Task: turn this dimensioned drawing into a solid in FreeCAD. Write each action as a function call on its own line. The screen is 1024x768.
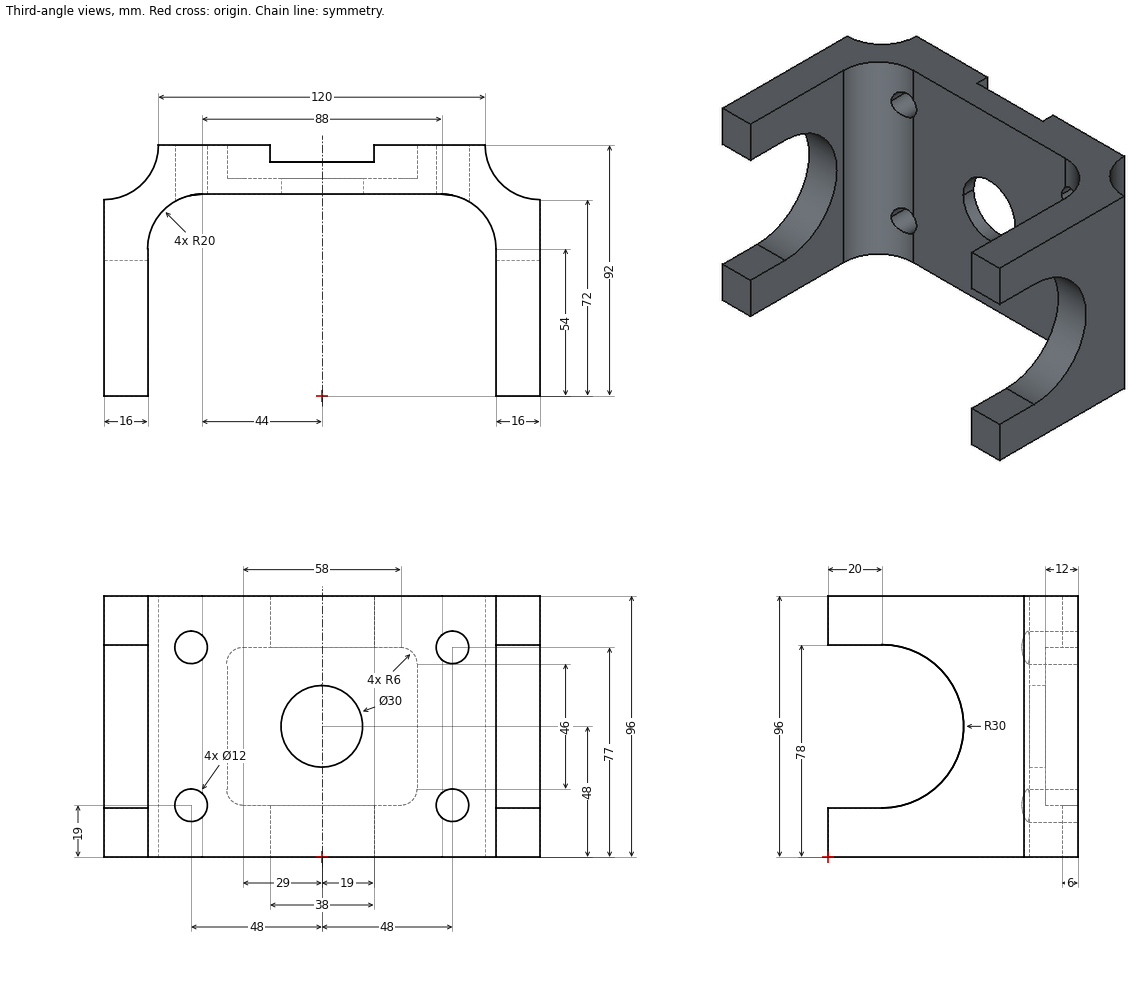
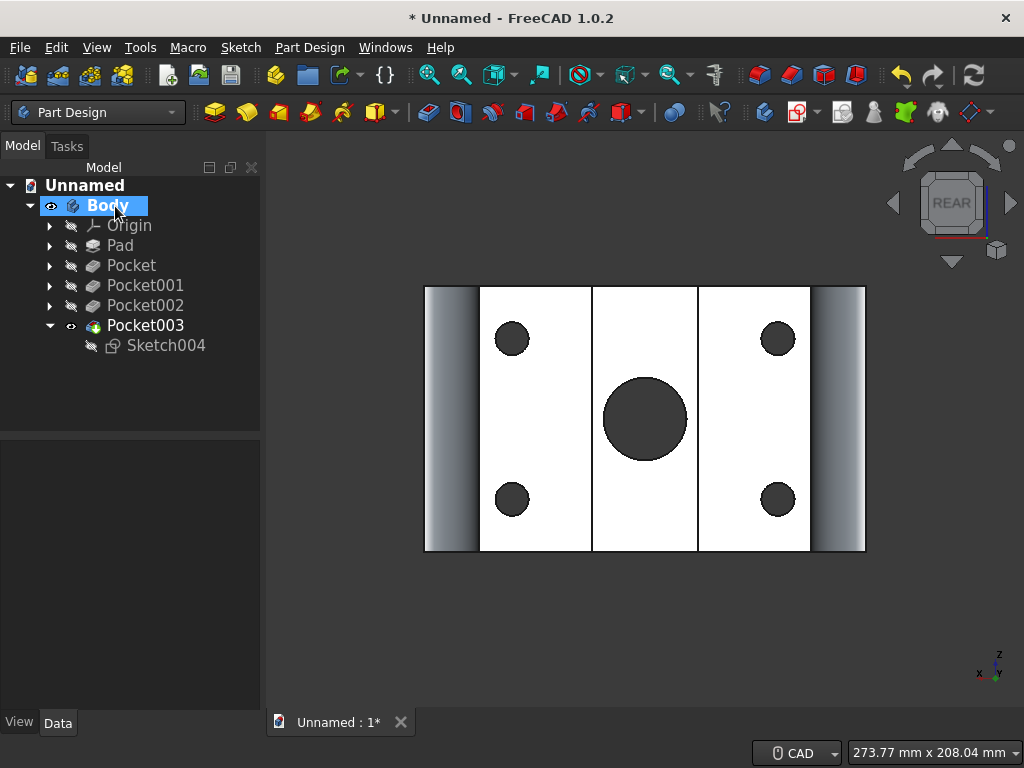
click(536, 418)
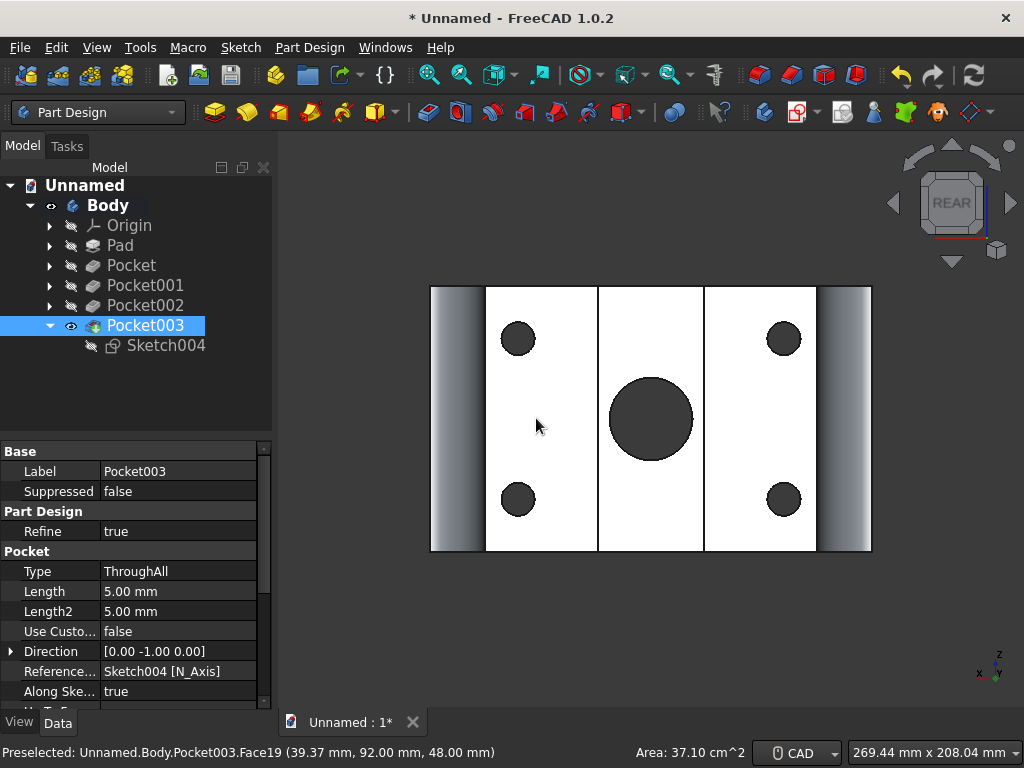
click(798, 112)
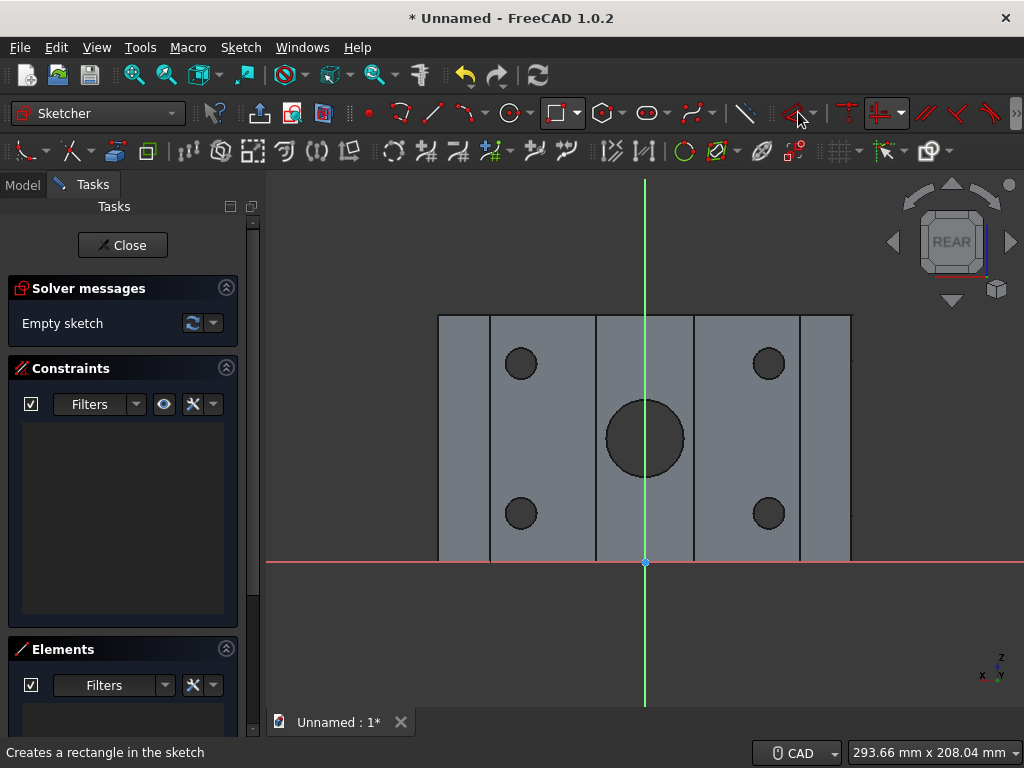
scroll(728, 493, up, 3)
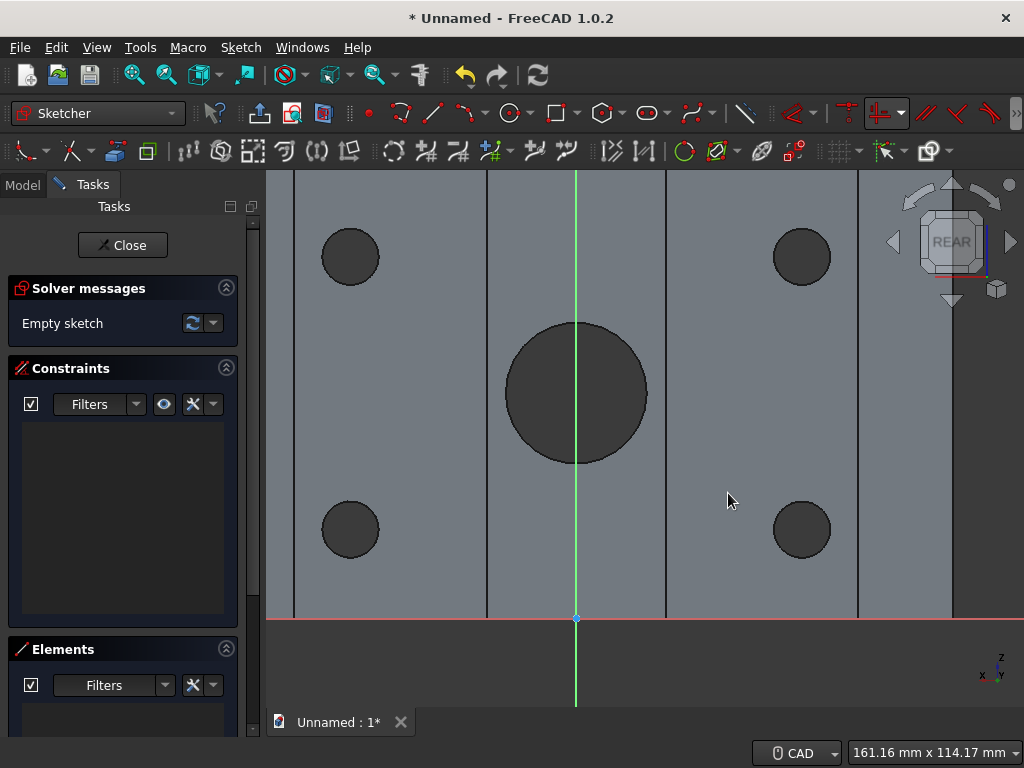
click(434, 114)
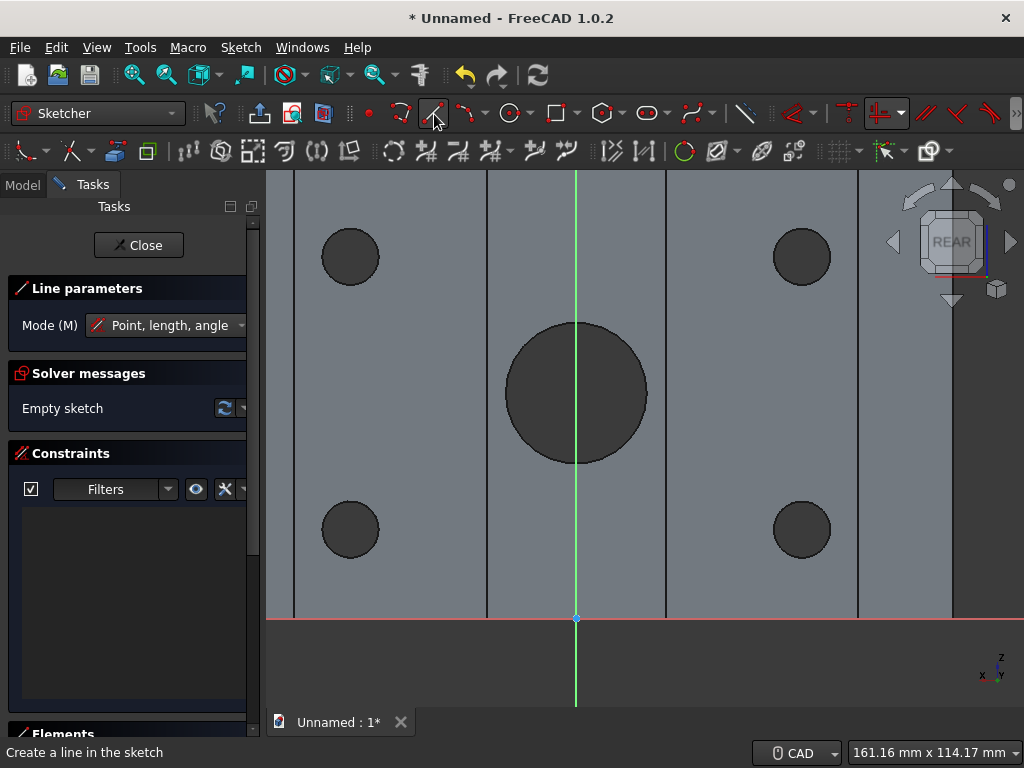
click(713, 257)
click(440, 257)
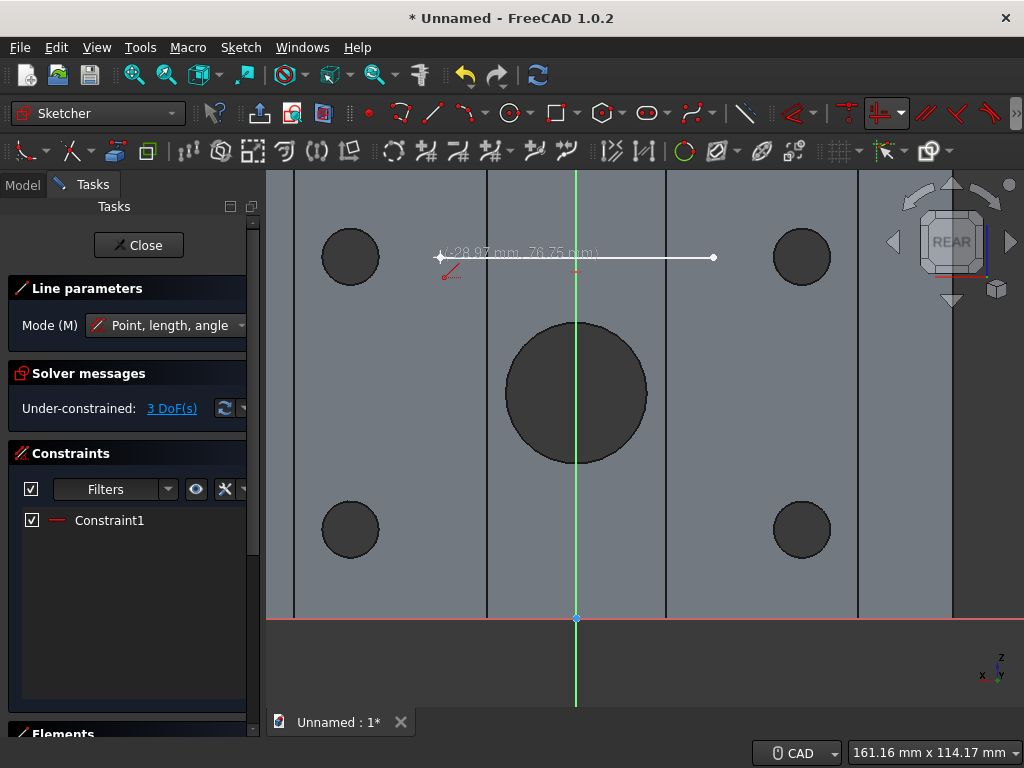
click(412, 285)
click(412, 501)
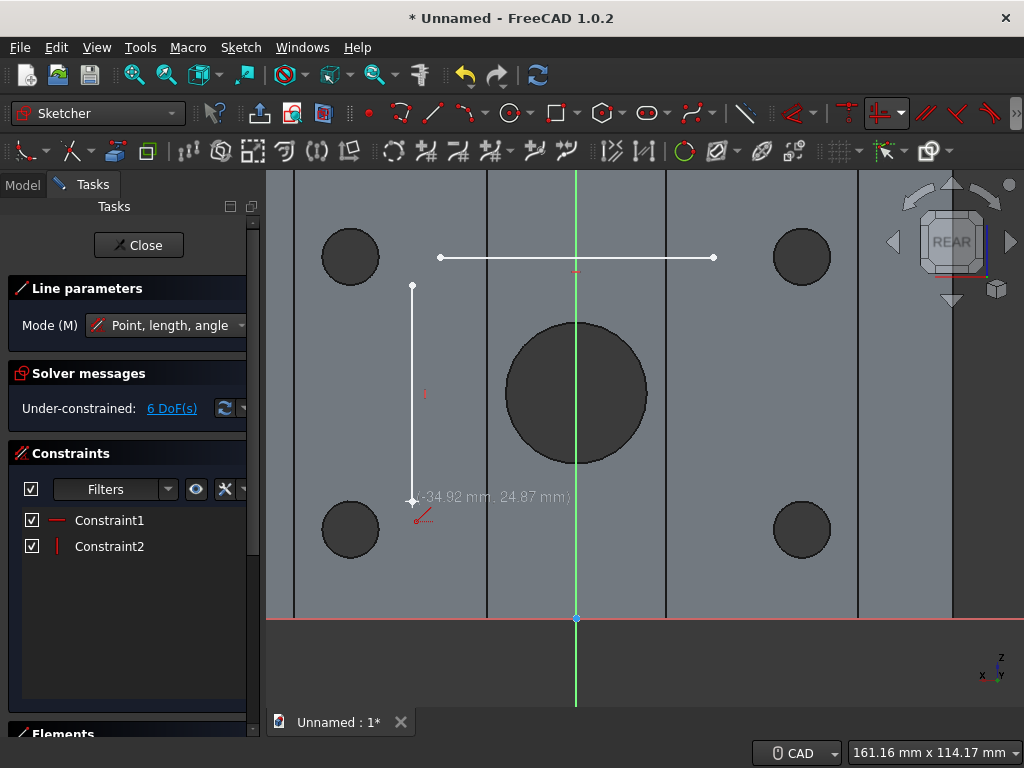
click(440, 530)
click(713, 530)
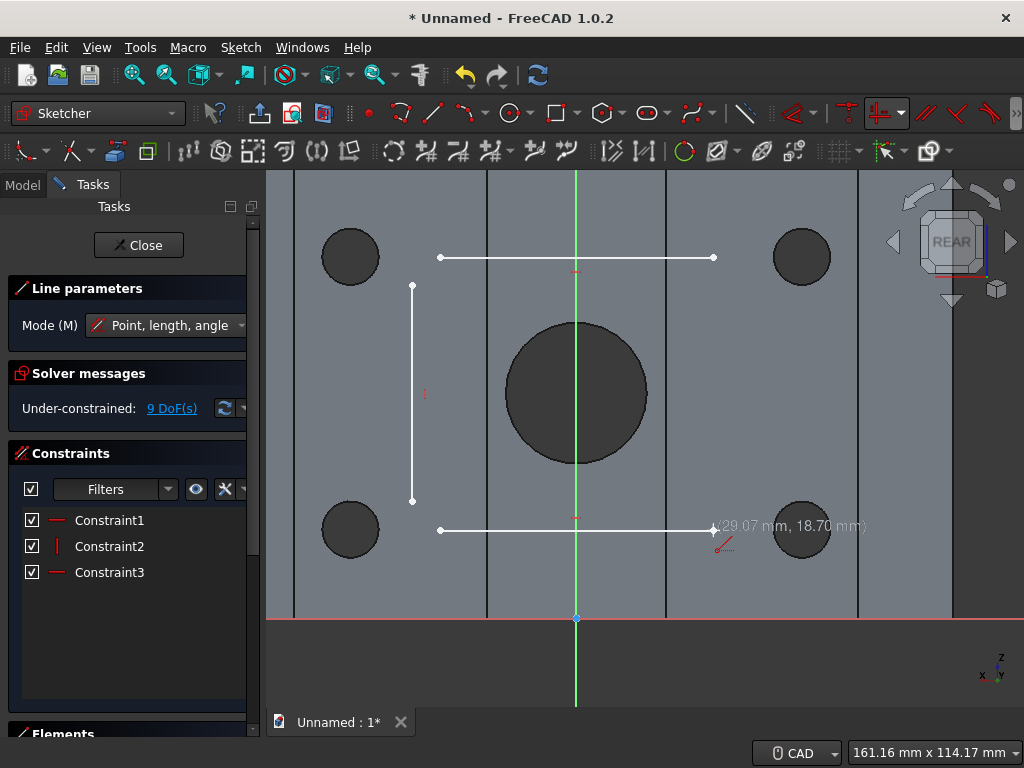
click(741, 501)
click(741, 285)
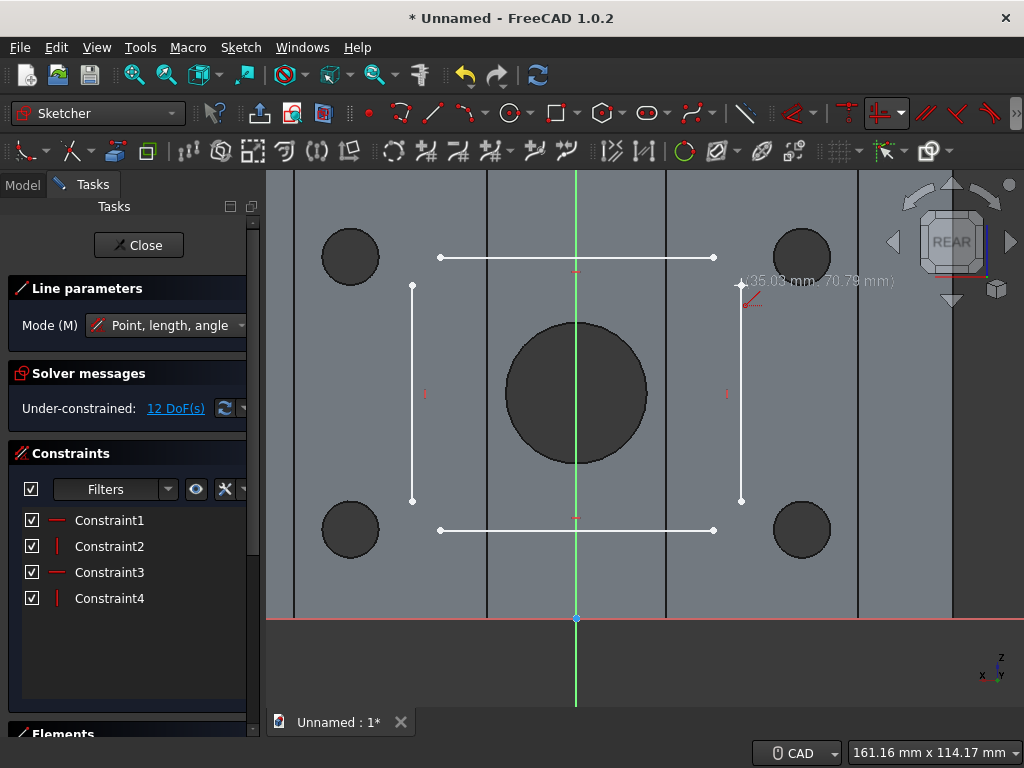
click(466, 114)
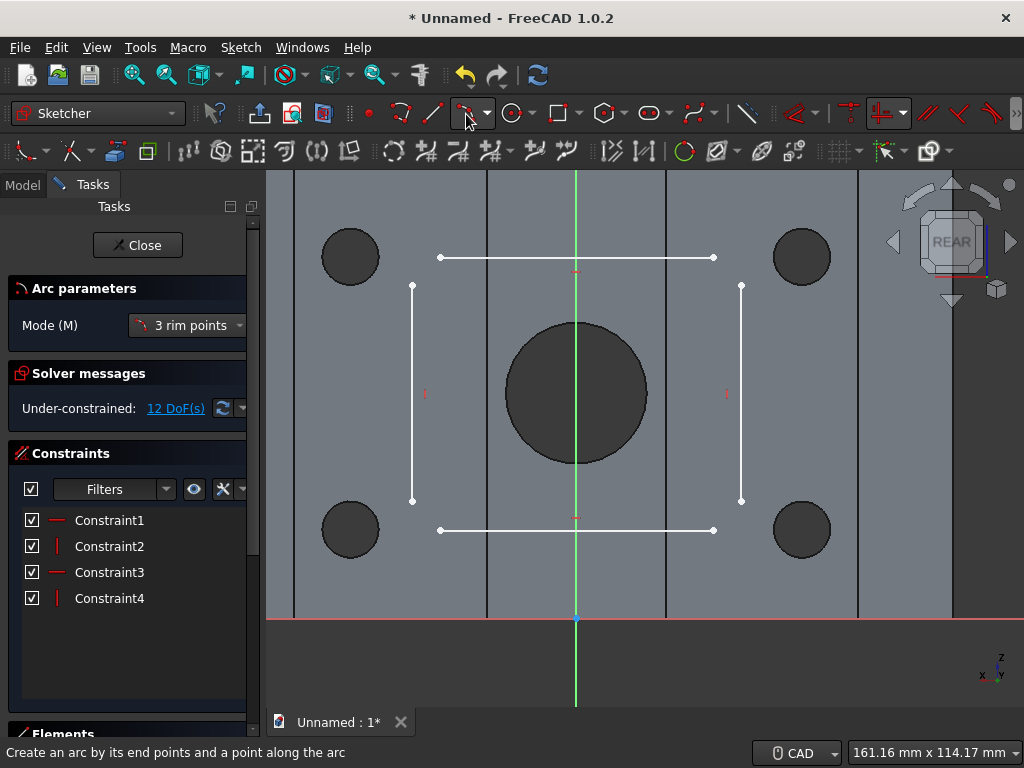
click(440, 258)
click(412, 286)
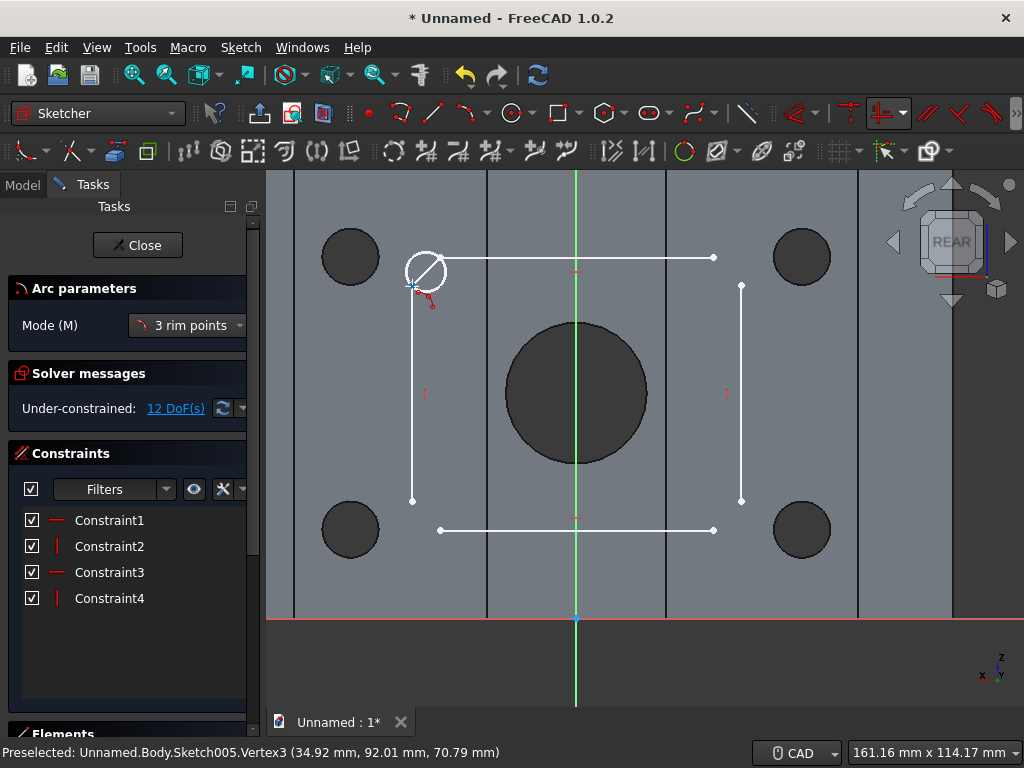
scroll(420, 265, up, 4)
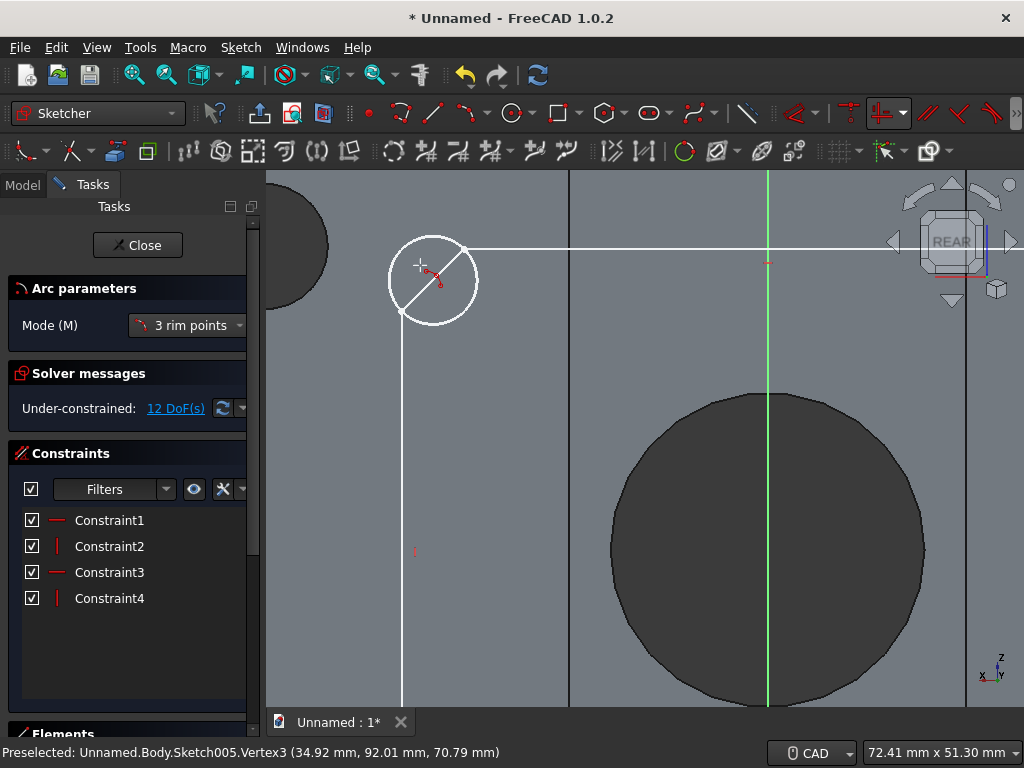
click(420, 265)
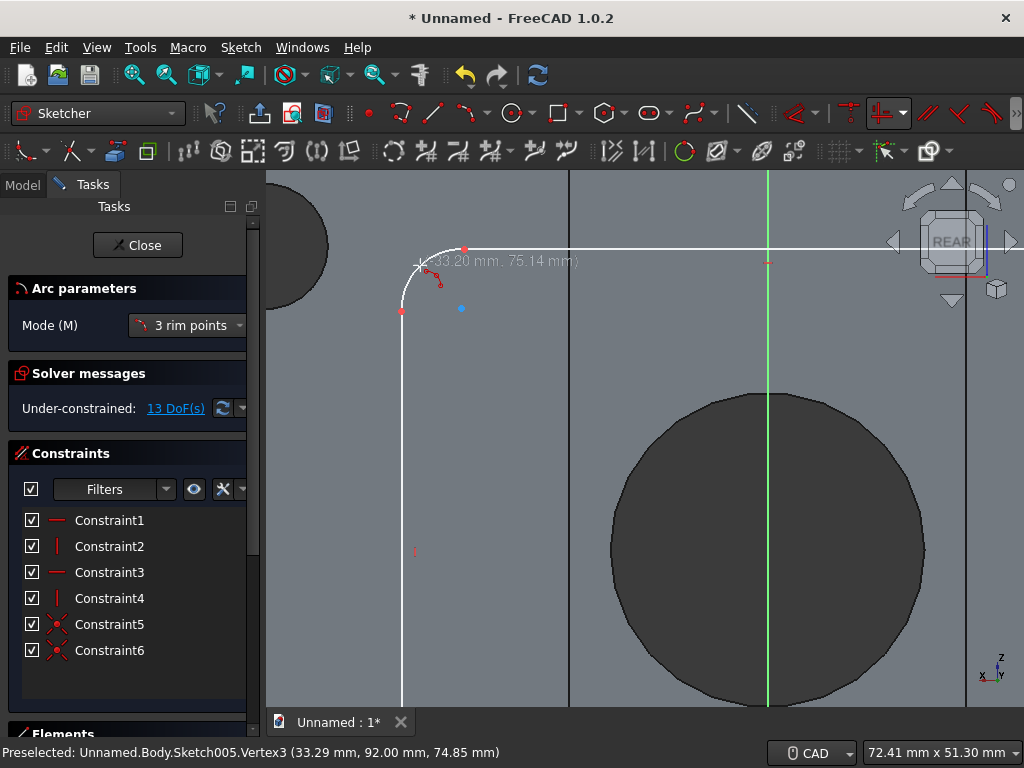
scroll(421, 266, down, 4)